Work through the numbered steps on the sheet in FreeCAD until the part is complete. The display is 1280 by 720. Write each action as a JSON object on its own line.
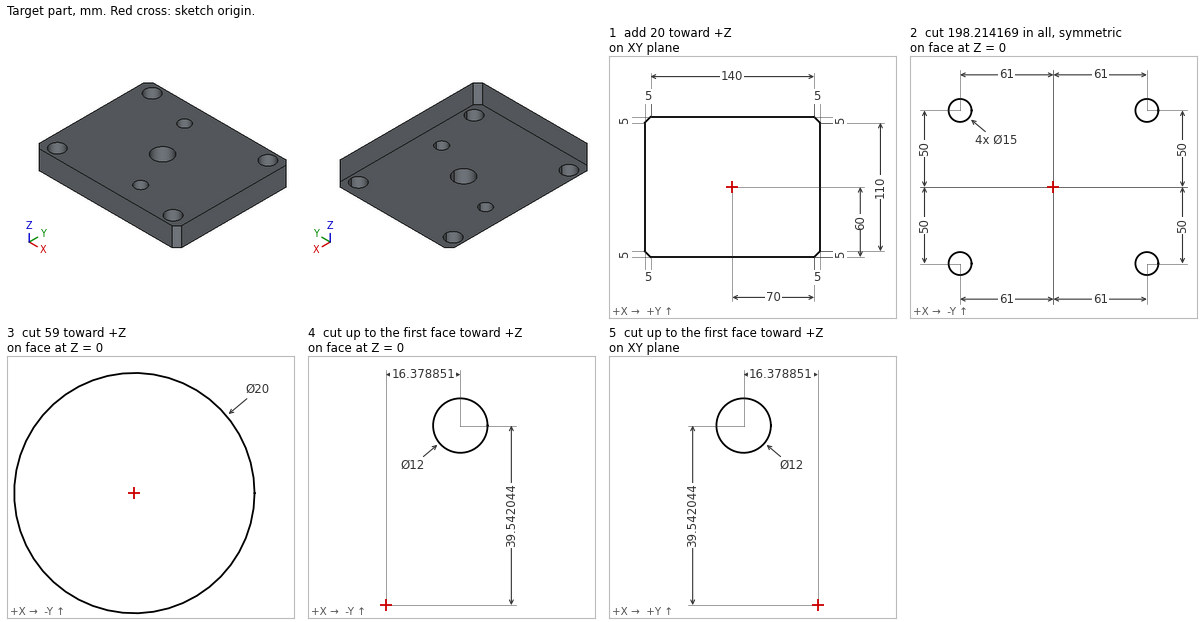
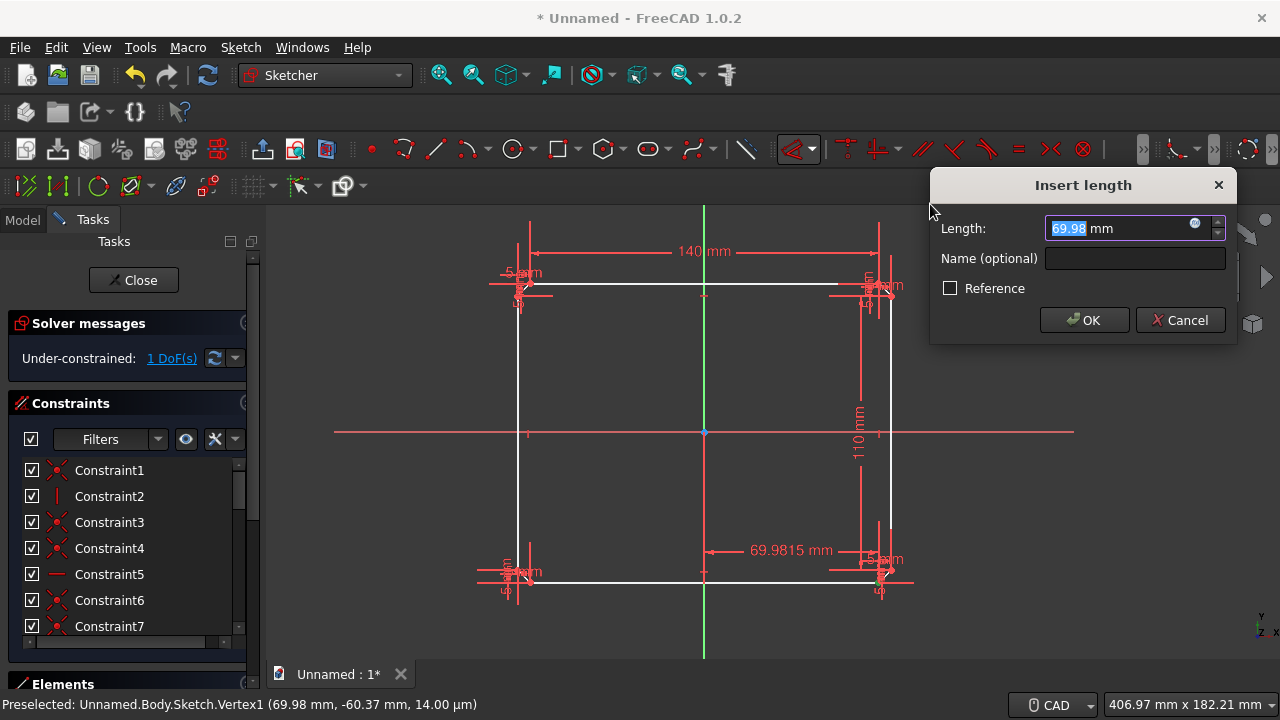
{"action": "type", "text": "70"}
{"action": "key", "text": "Return"}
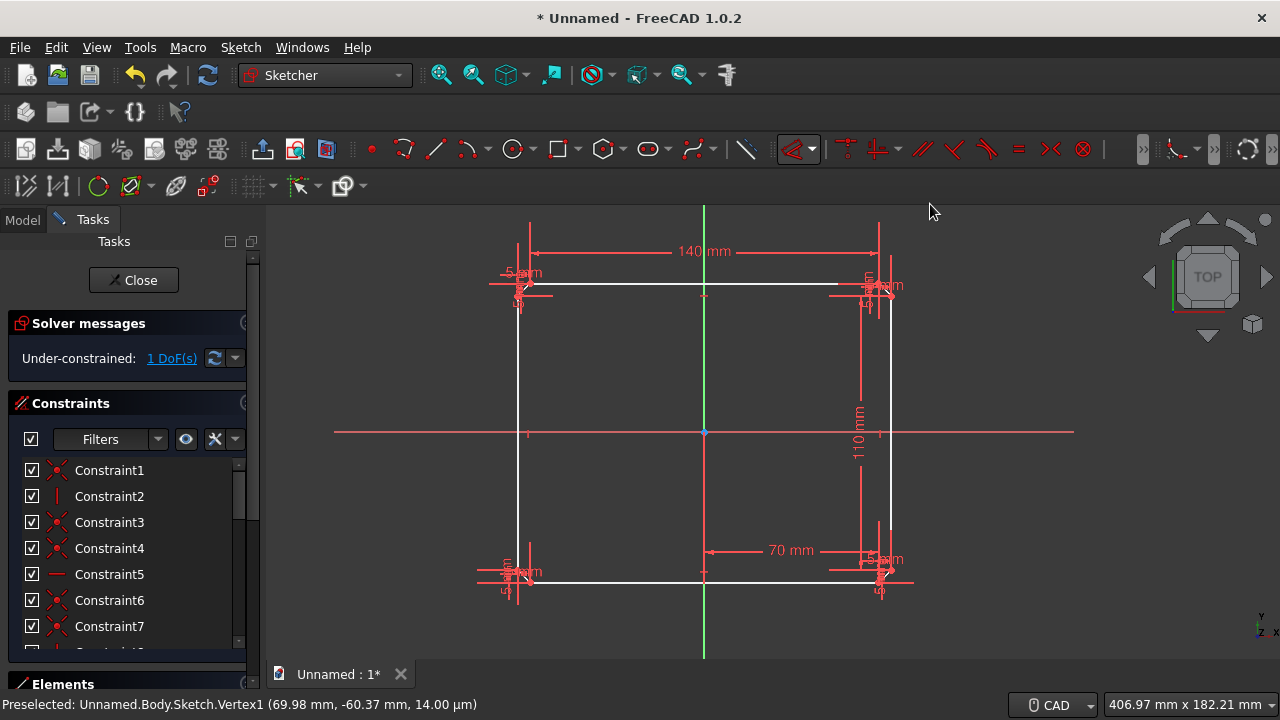
{"action": "left_click", "coordinate": [879, 583]}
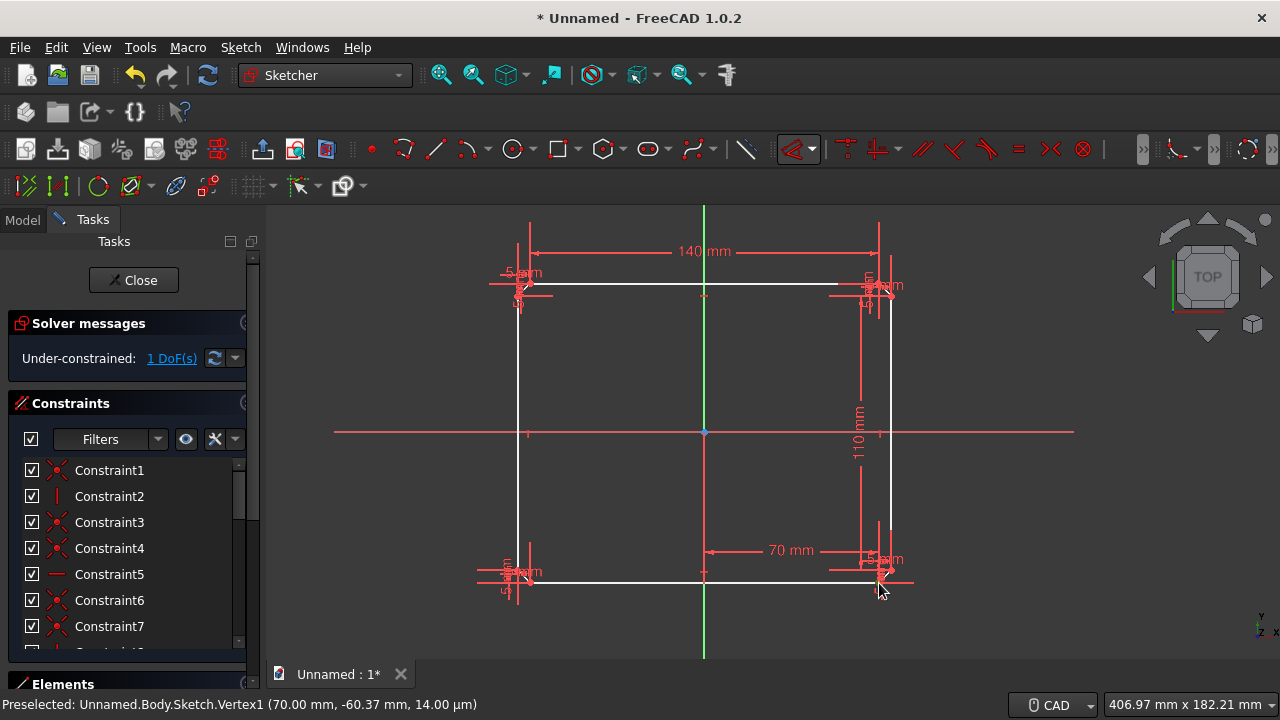
{"action": "left_click", "coordinate": [814, 150]}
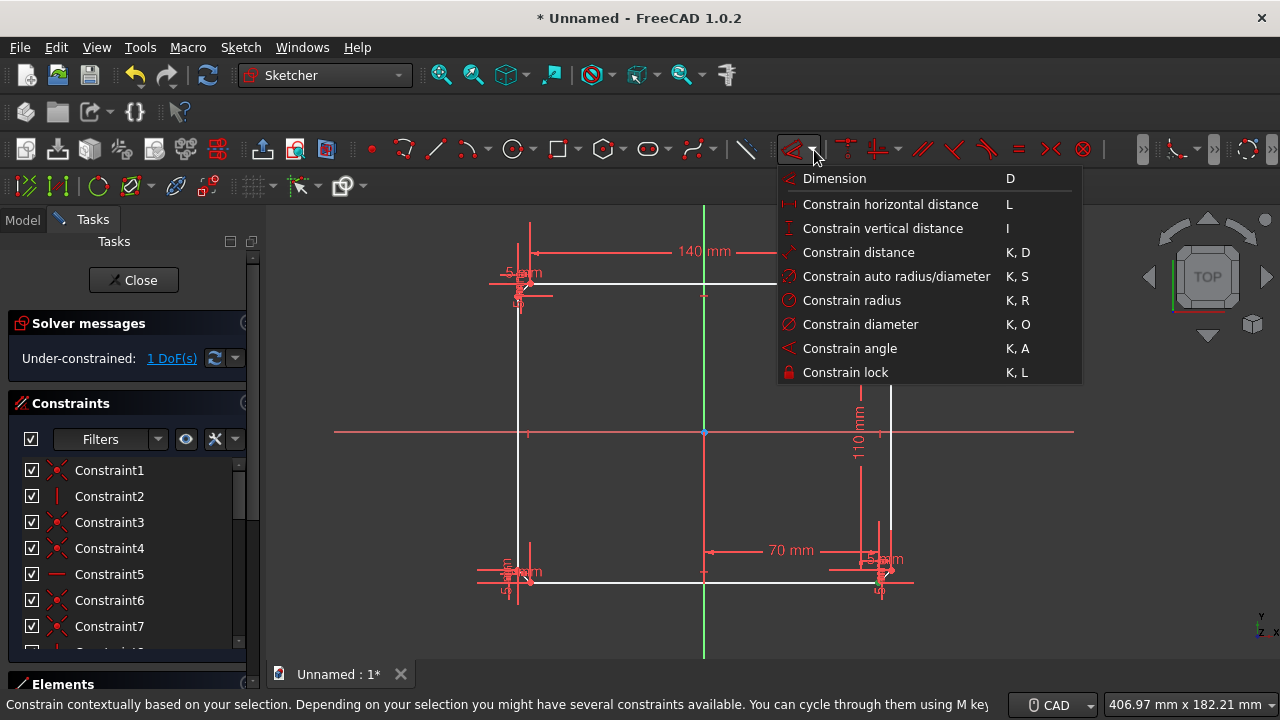
{"action": "left_click", "coordinate": [930, 228]}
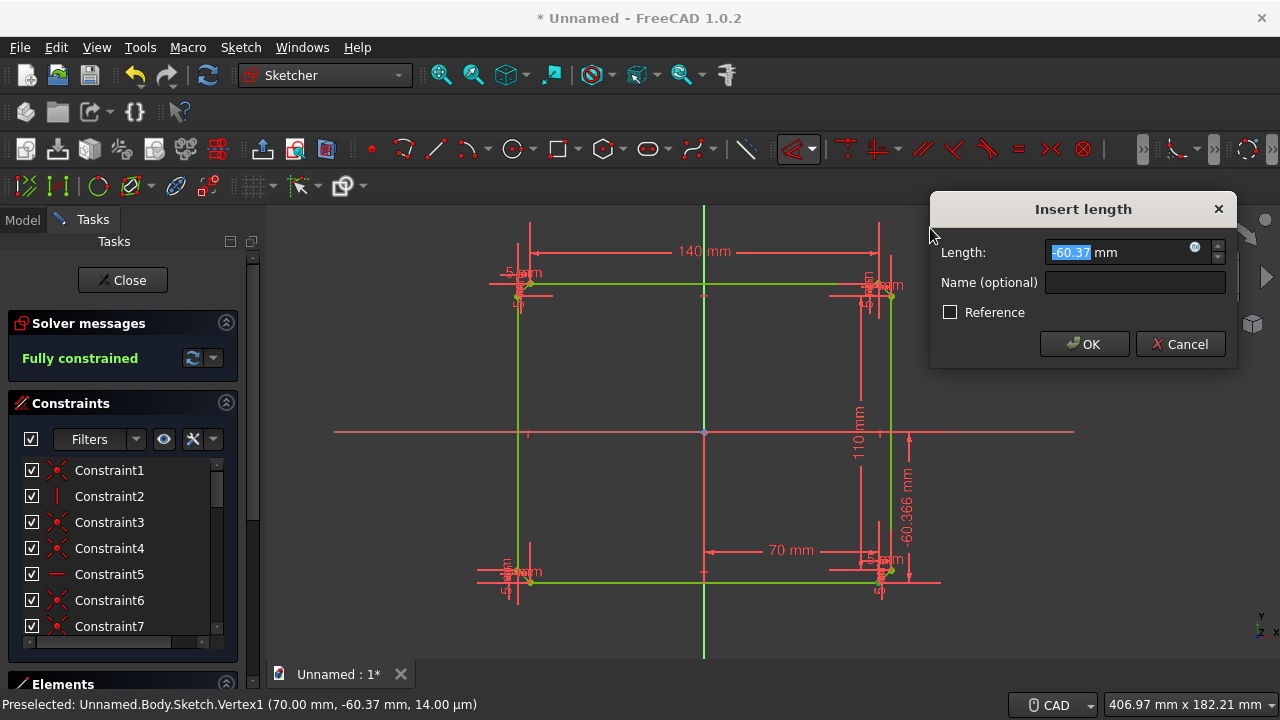
{"action": "type", "text": "-60"}
{"action": "key", "text": "Return"}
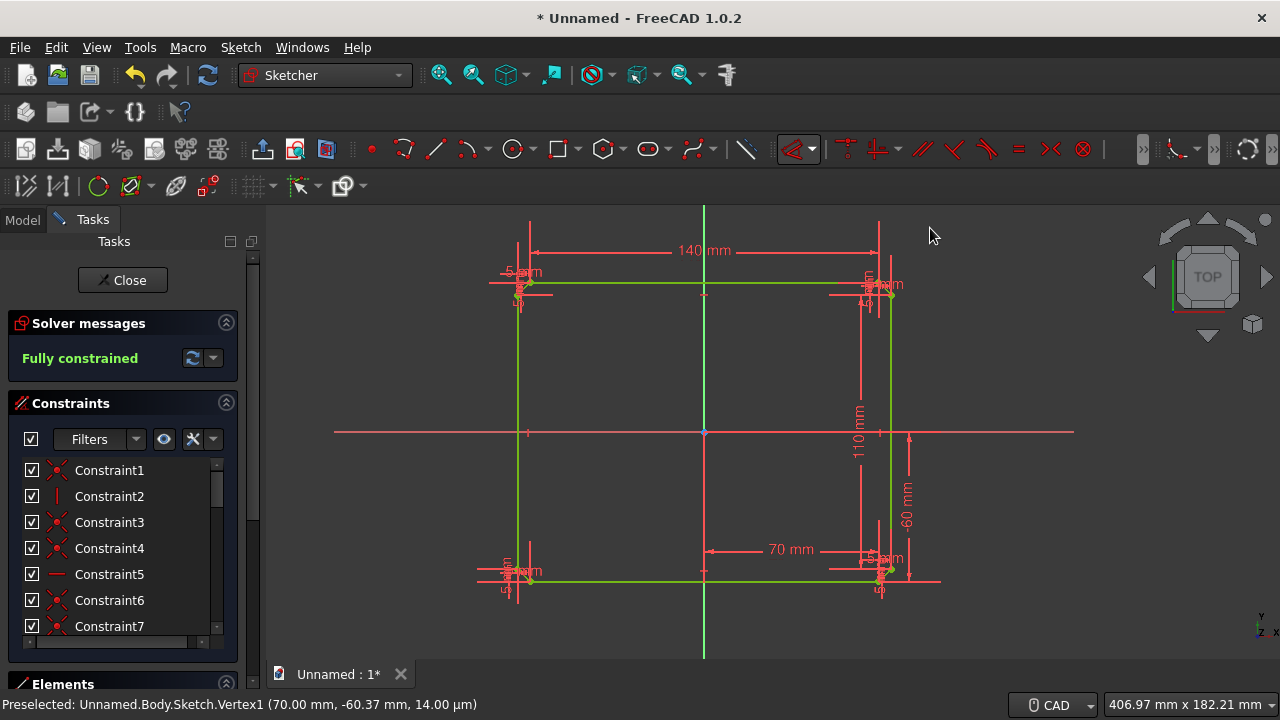
{"action": "left_click", "coordinate": [123, 280]}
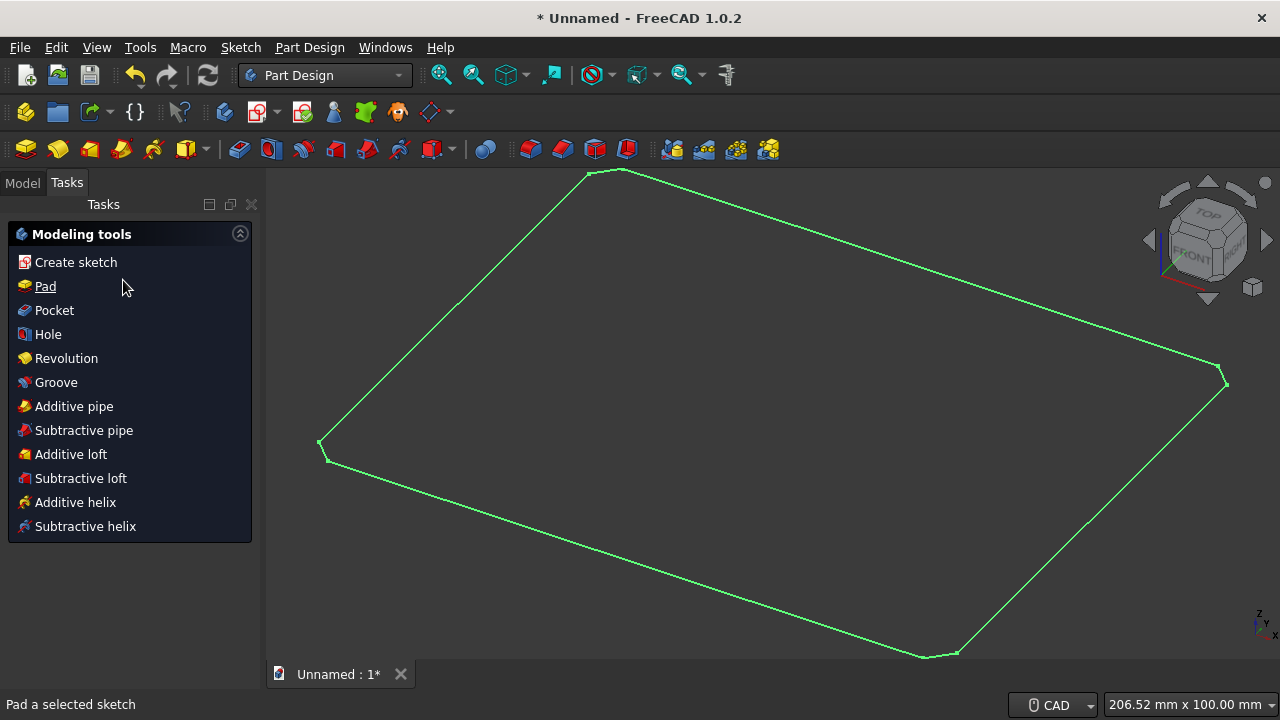
{"action": "left_click", "coordinate": [26, 150]}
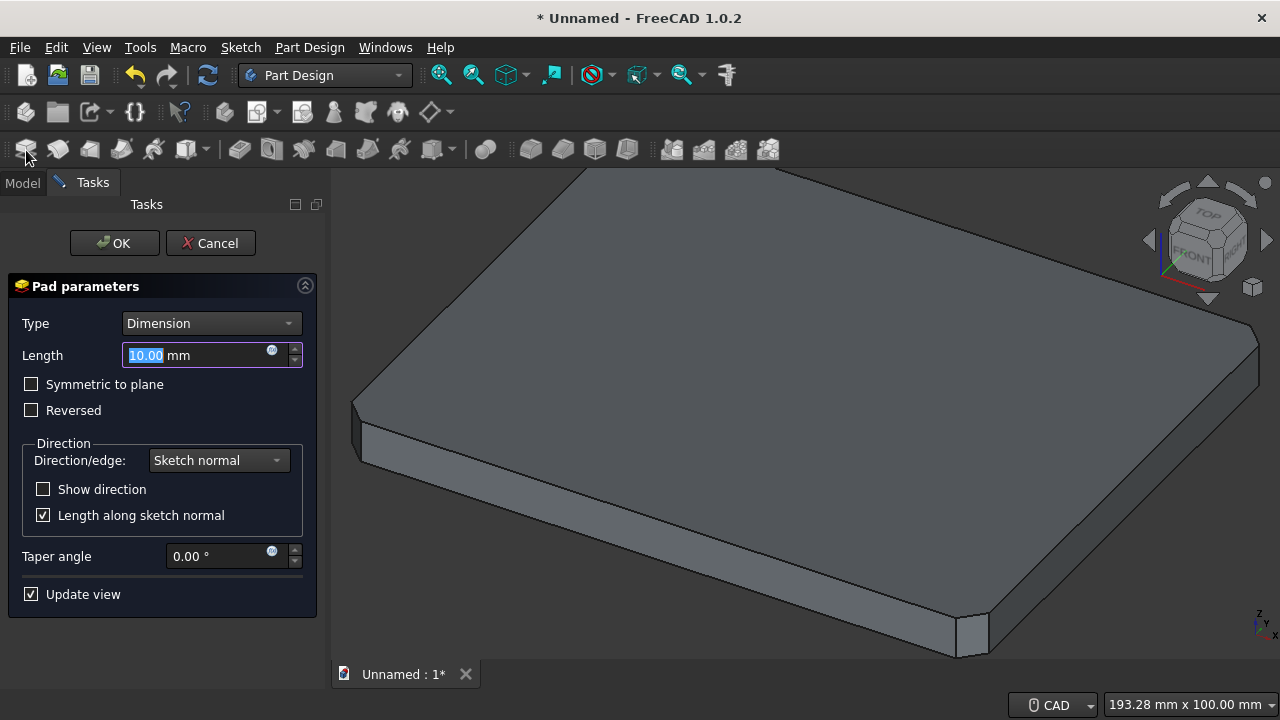
{"action": "type", "text": "20"}
{"action": "key", "text": "Tab"}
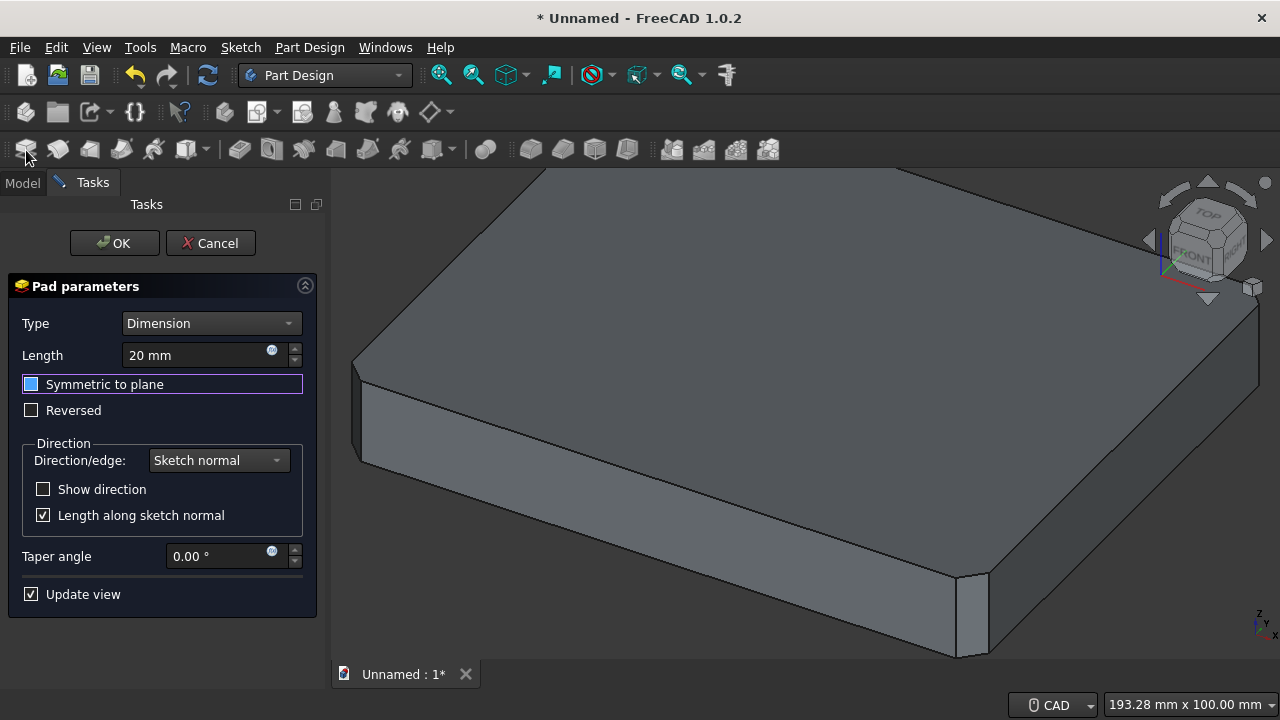
{"action": "left_click", "coordinate": [115, 243]}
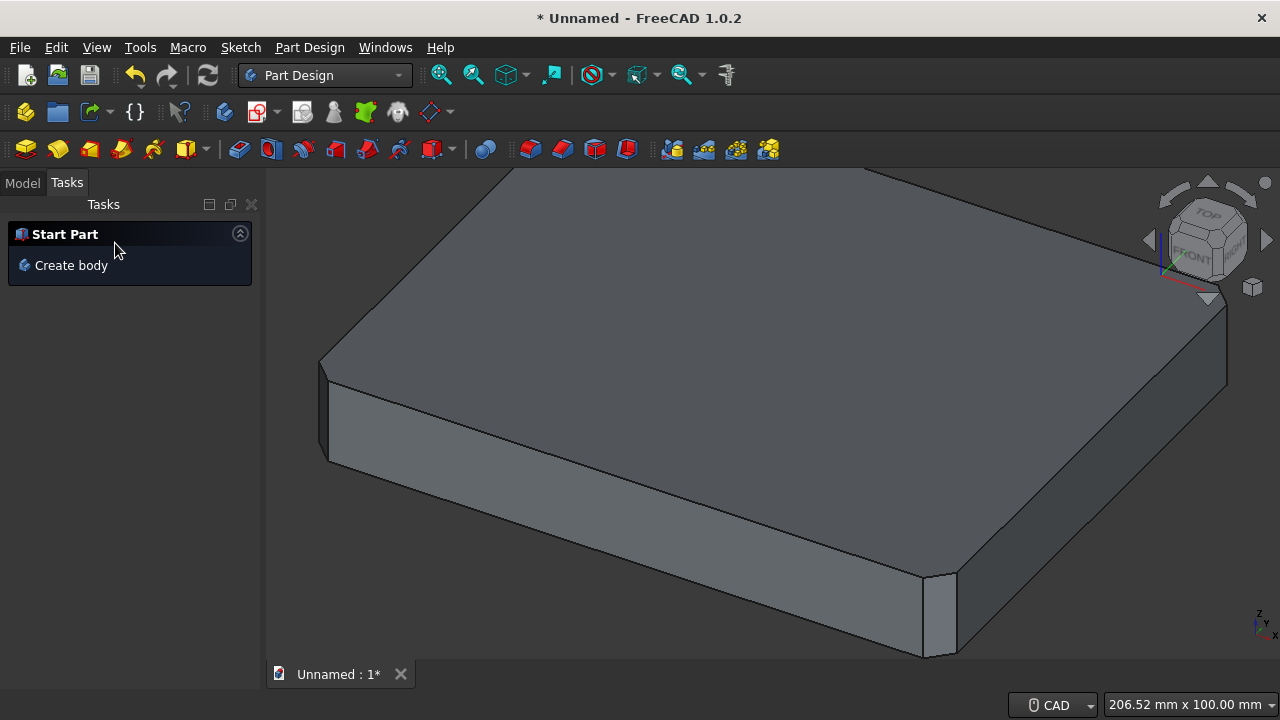
{"action": "key", "text": "v f"}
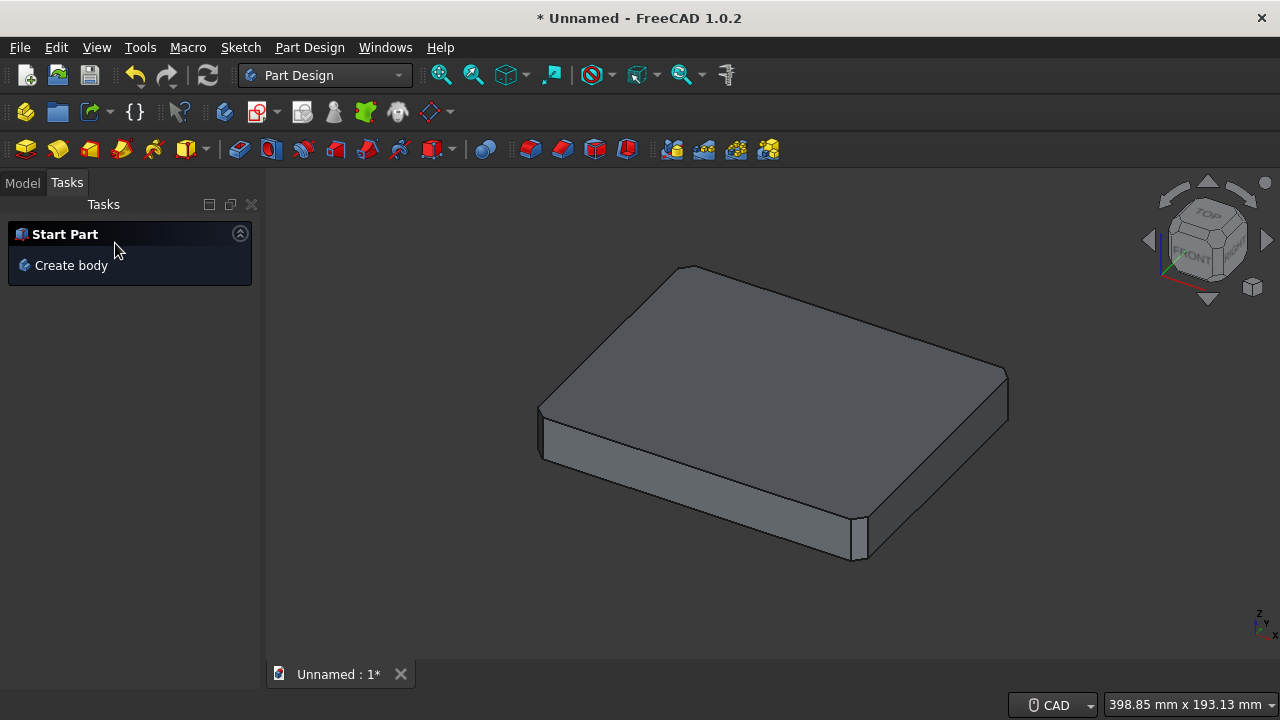
{"action": "key", "text": "5"}